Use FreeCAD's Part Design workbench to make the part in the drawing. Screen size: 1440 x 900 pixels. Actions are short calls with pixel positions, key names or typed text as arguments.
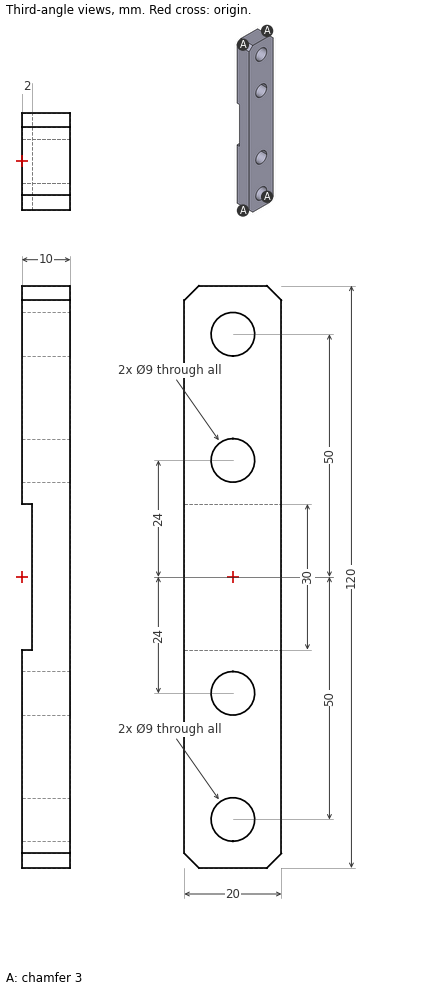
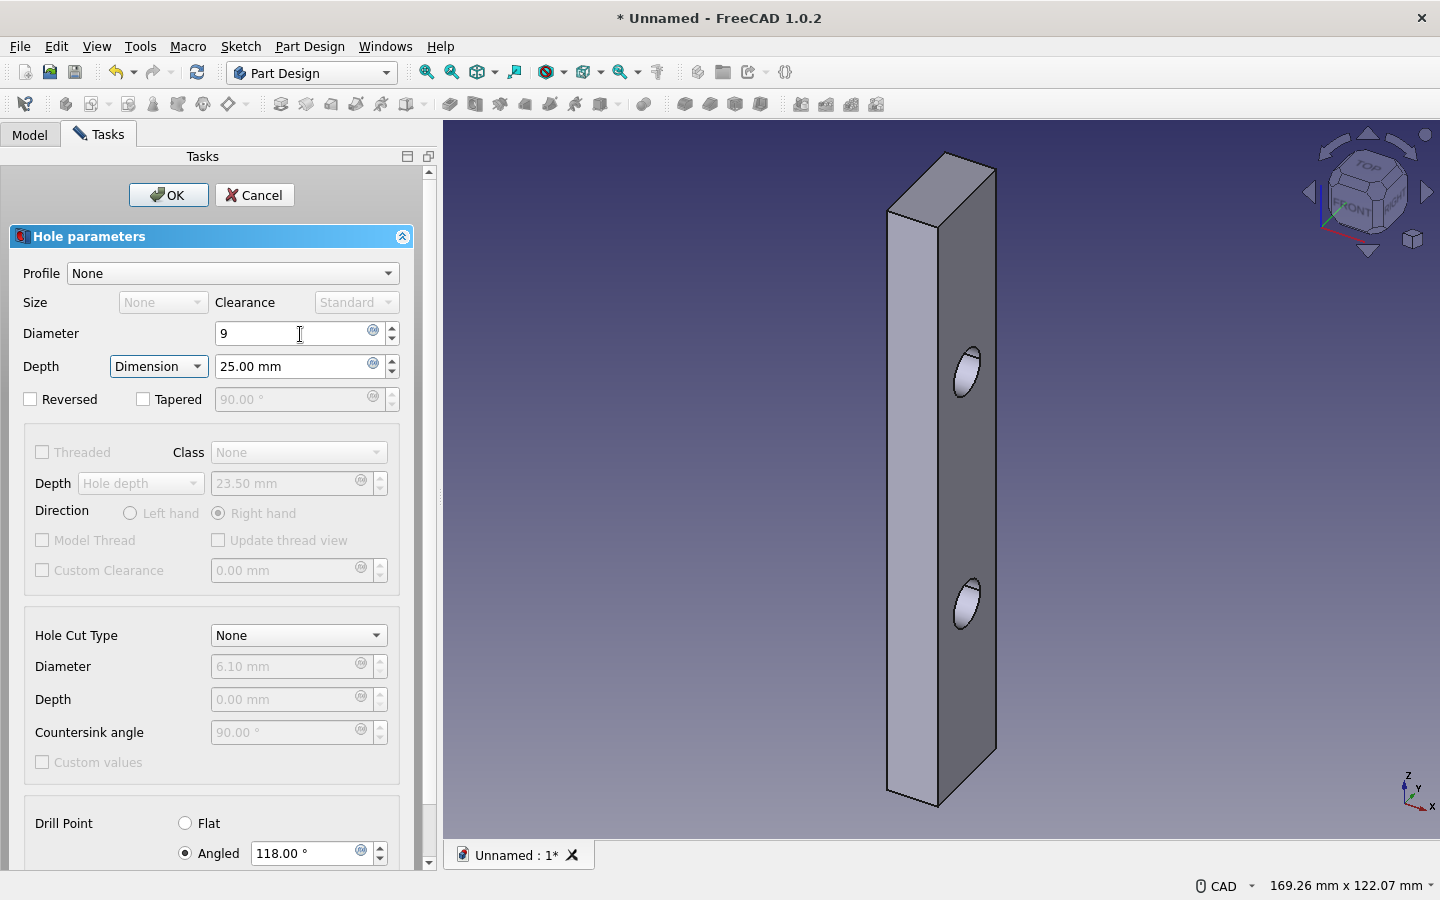
click(160, 366)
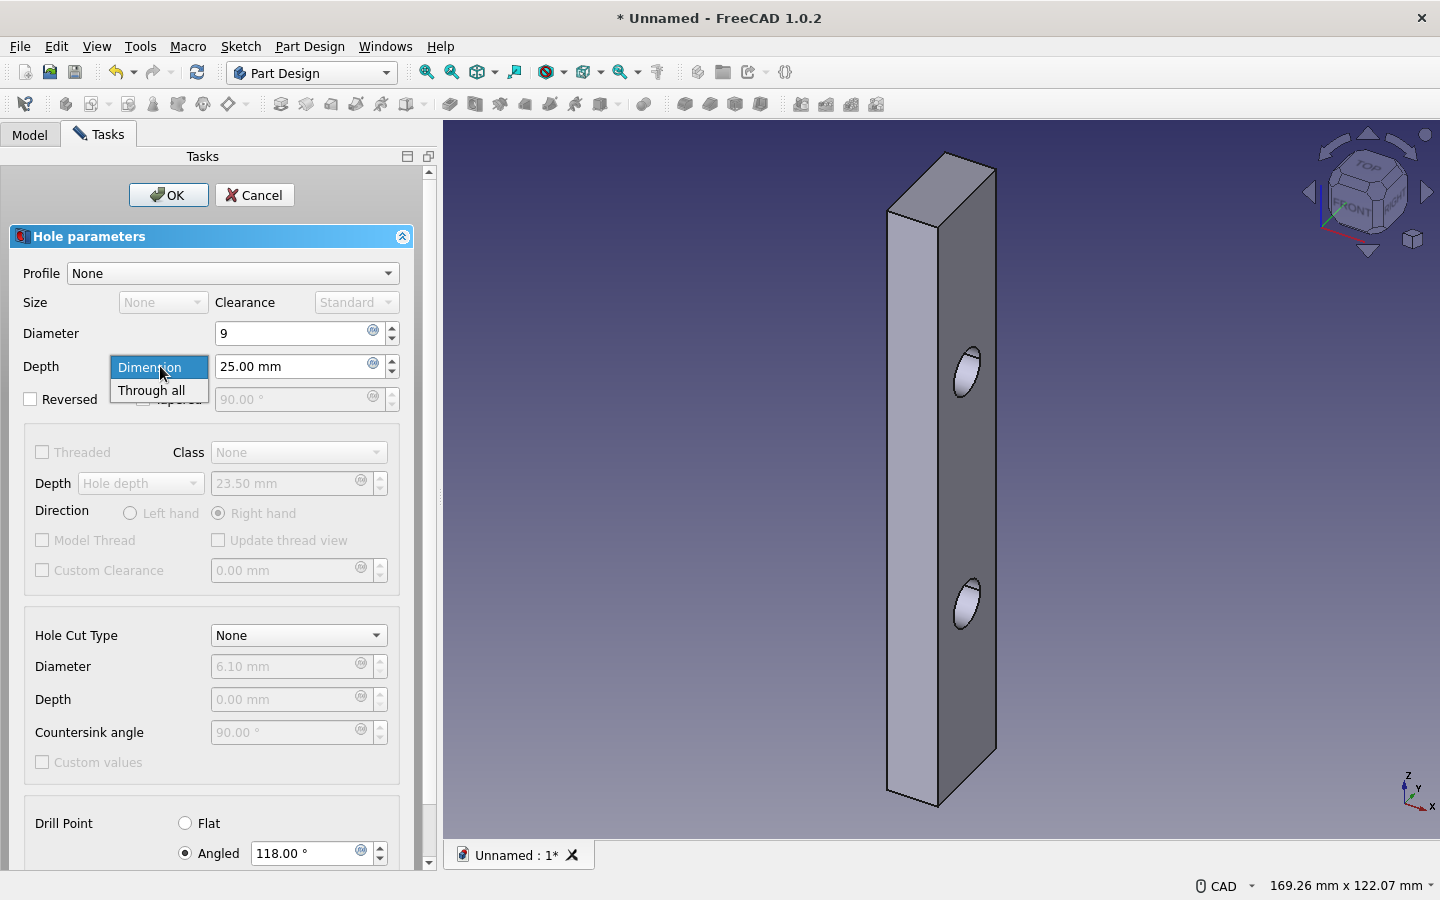
click(158, 390)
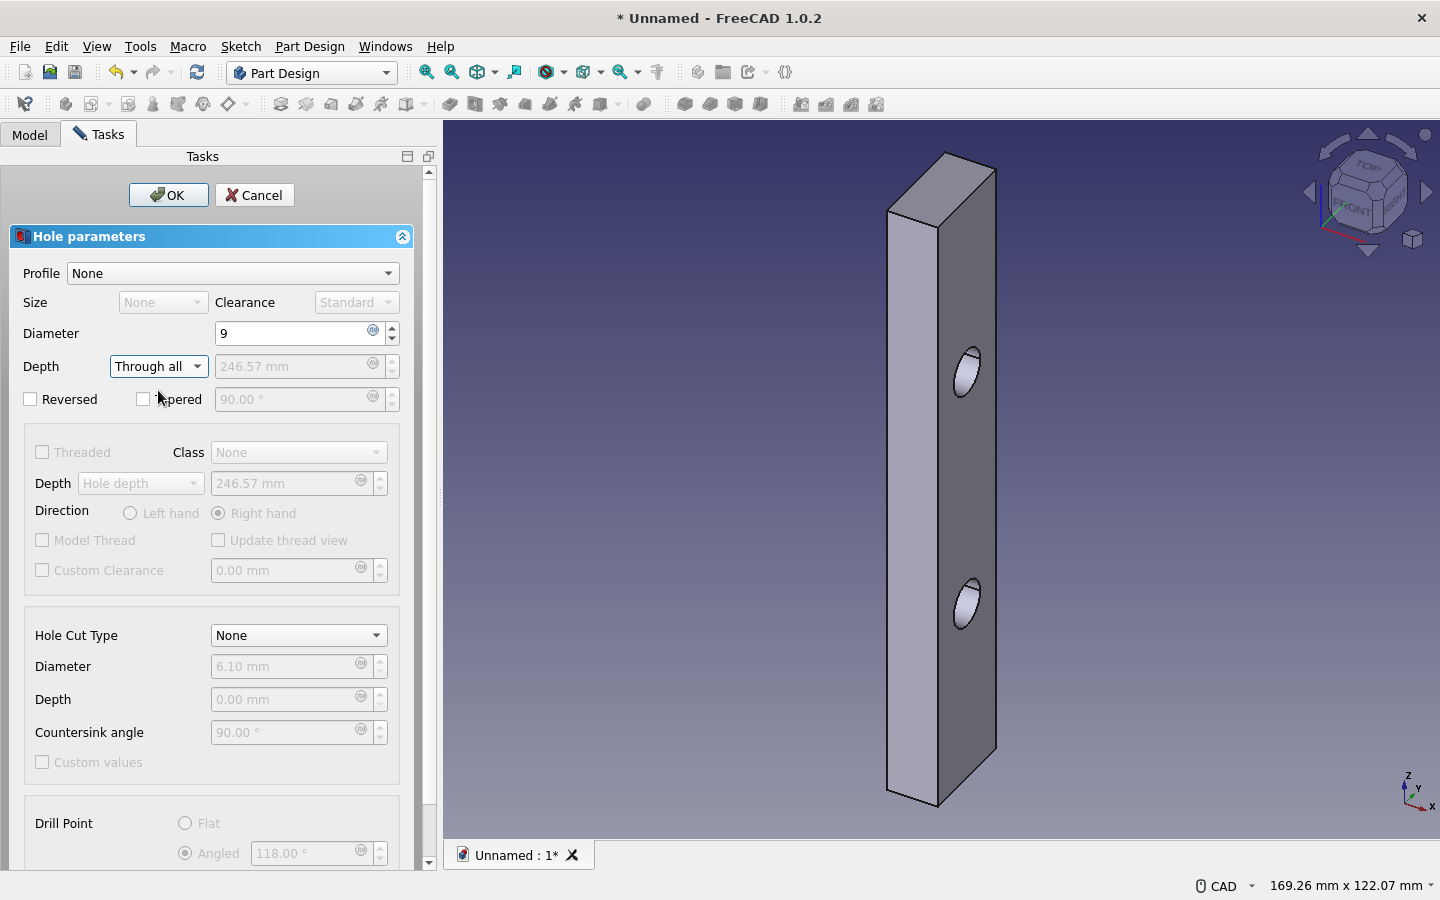
click(31, 399)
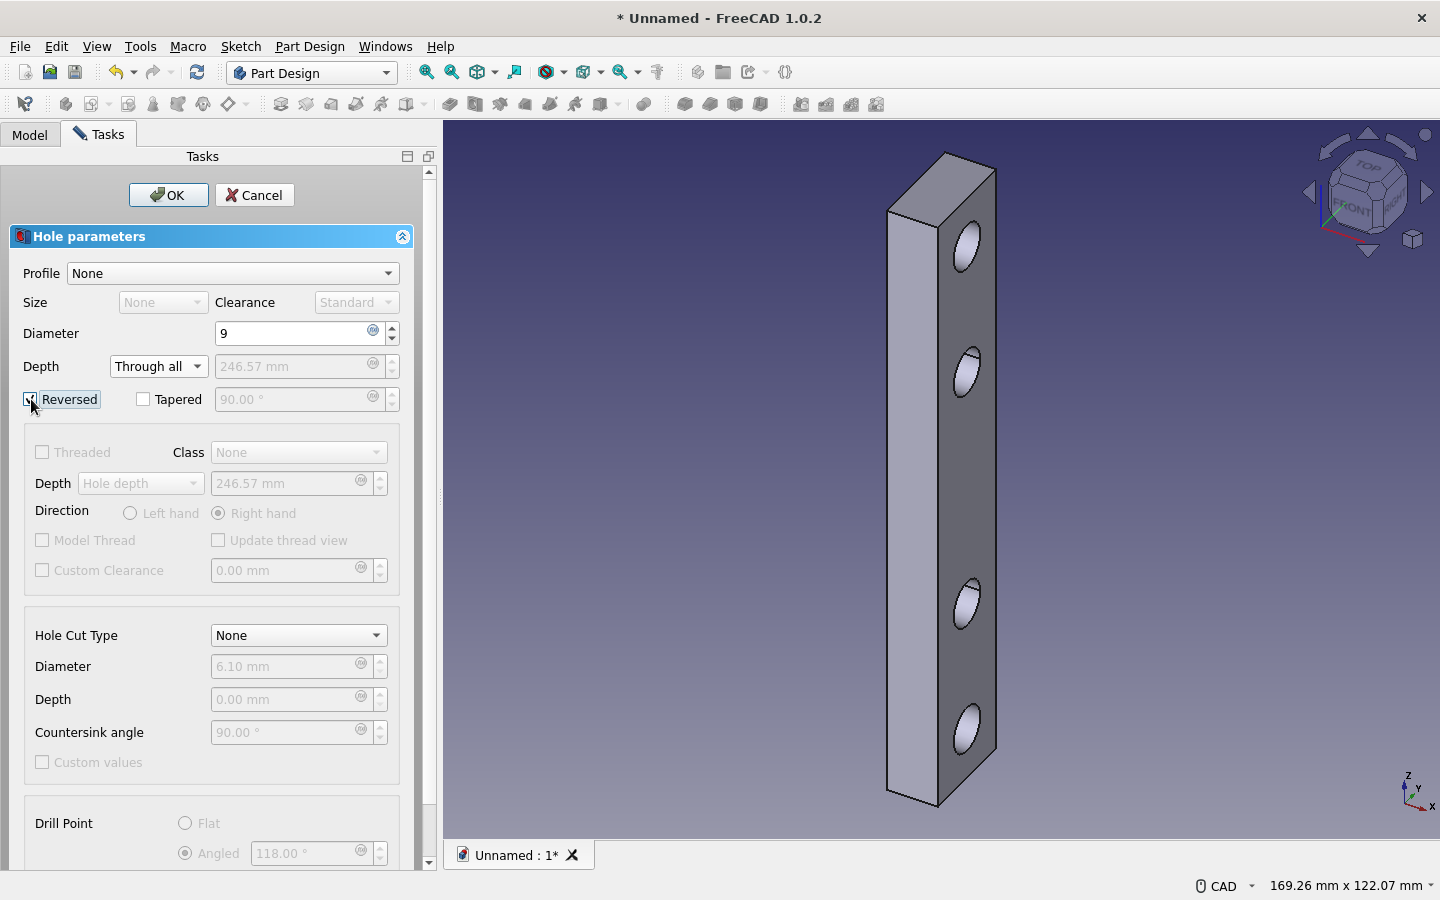
click(169, 195)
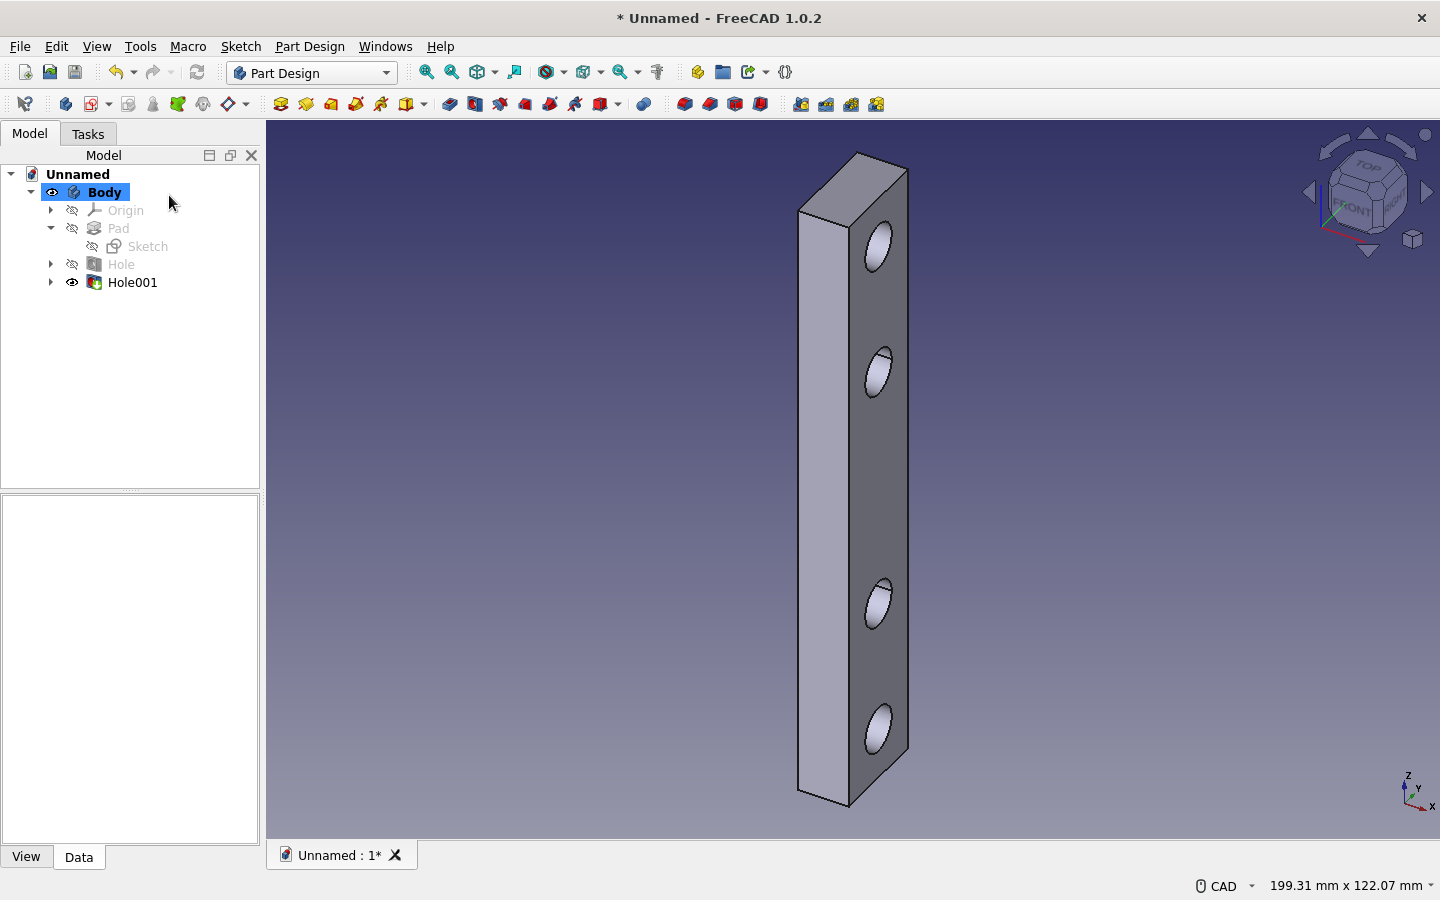
key(6)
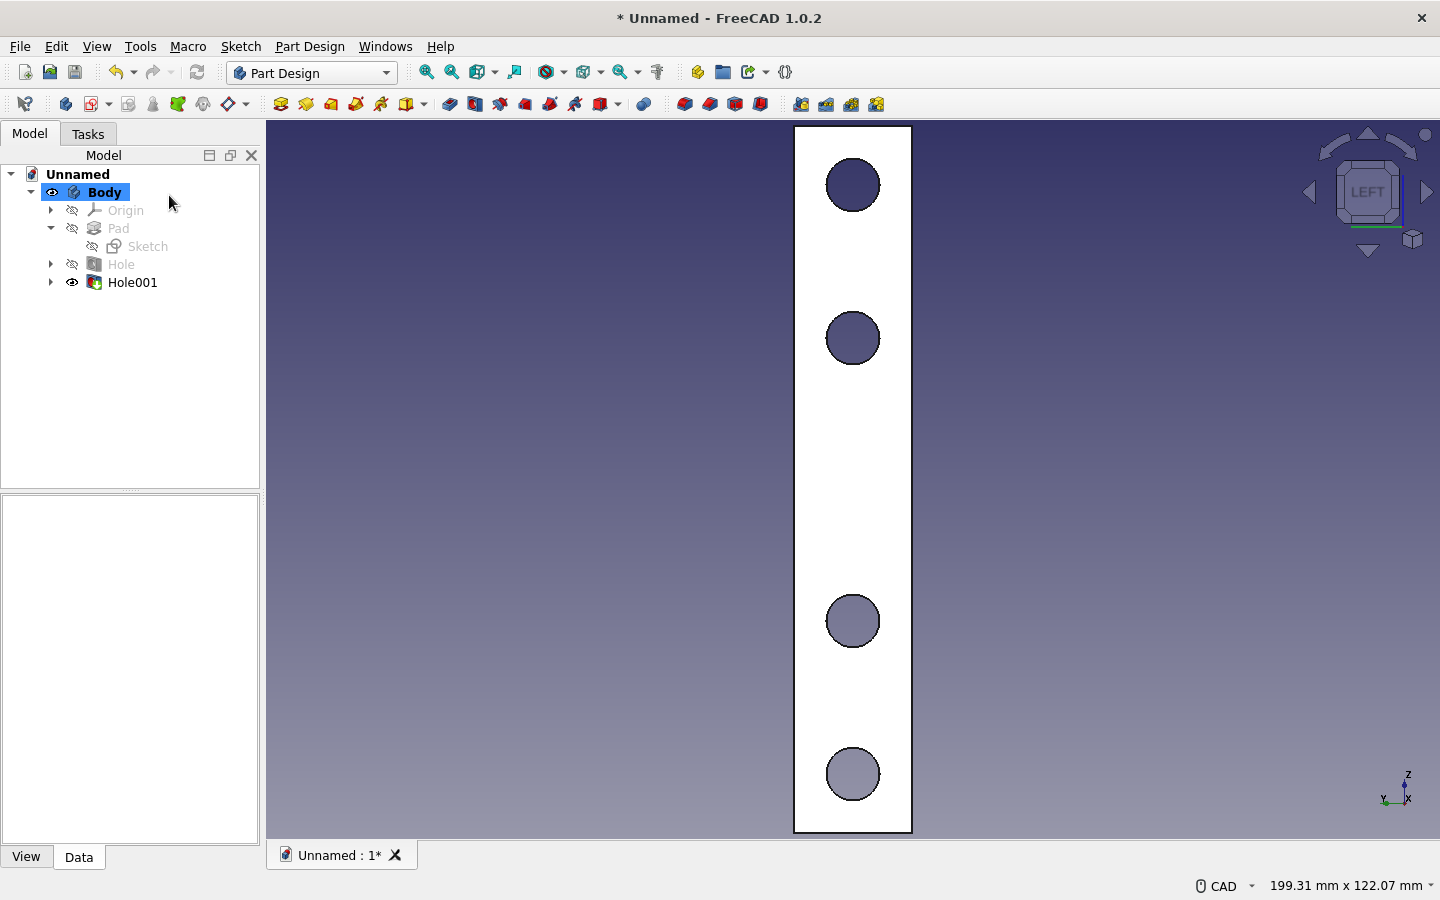
click(853, 478)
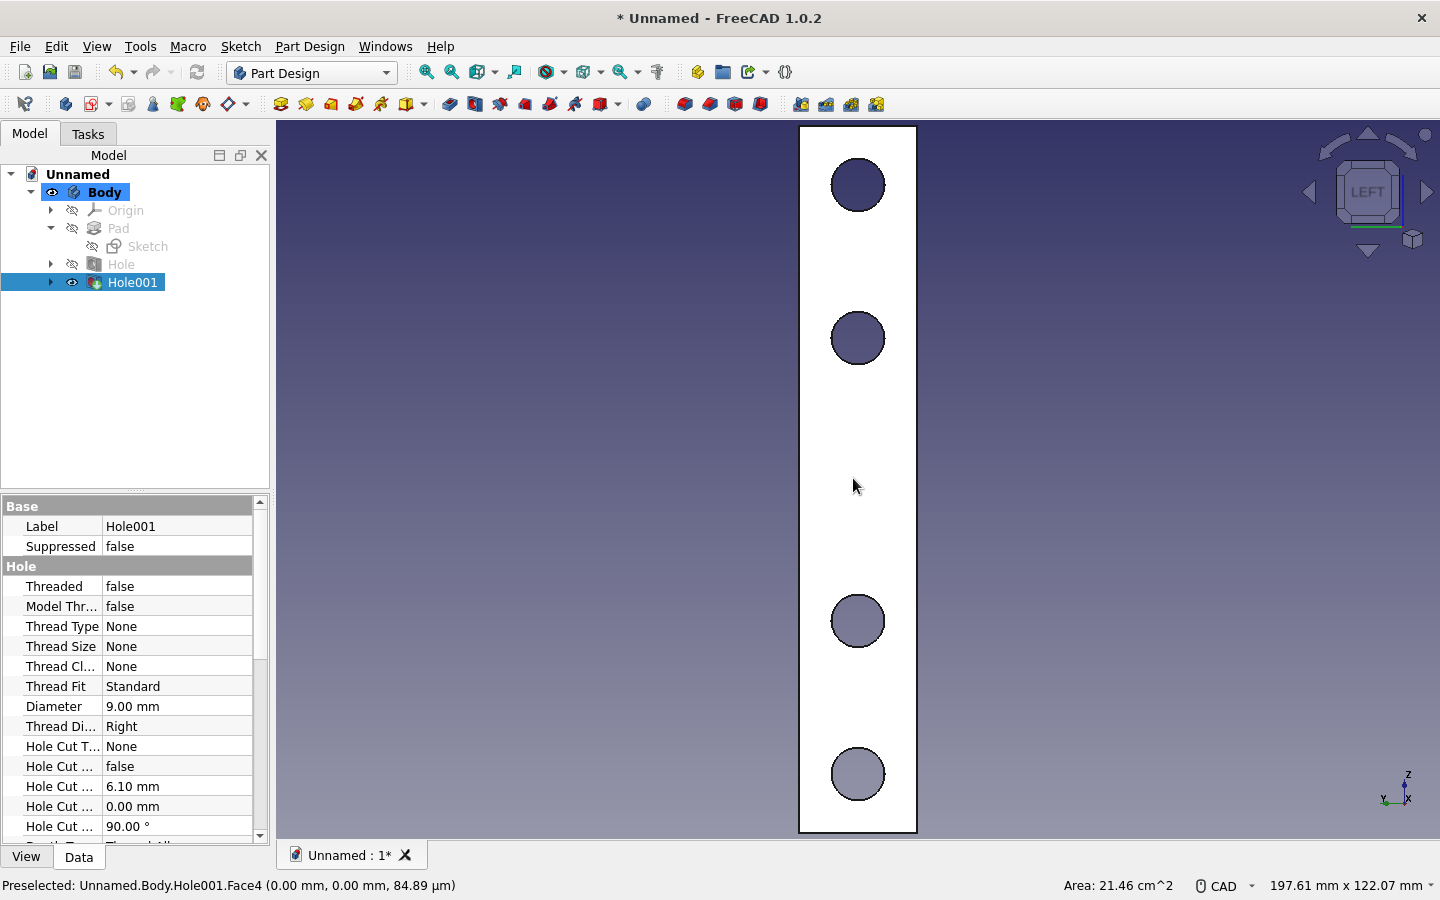
click(90, 104)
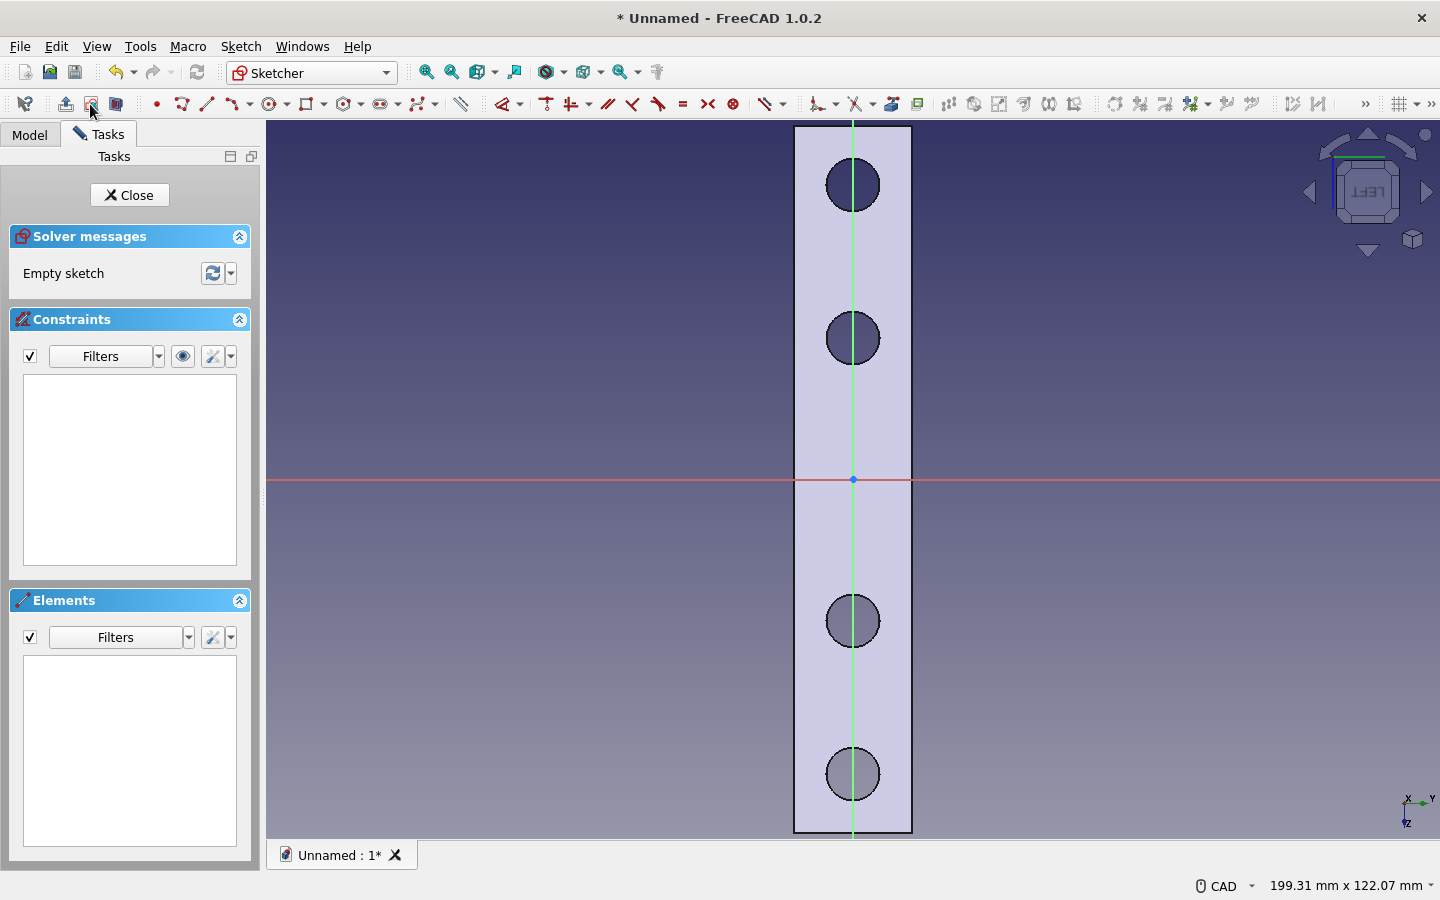
scroll(893, 480, up, 5)